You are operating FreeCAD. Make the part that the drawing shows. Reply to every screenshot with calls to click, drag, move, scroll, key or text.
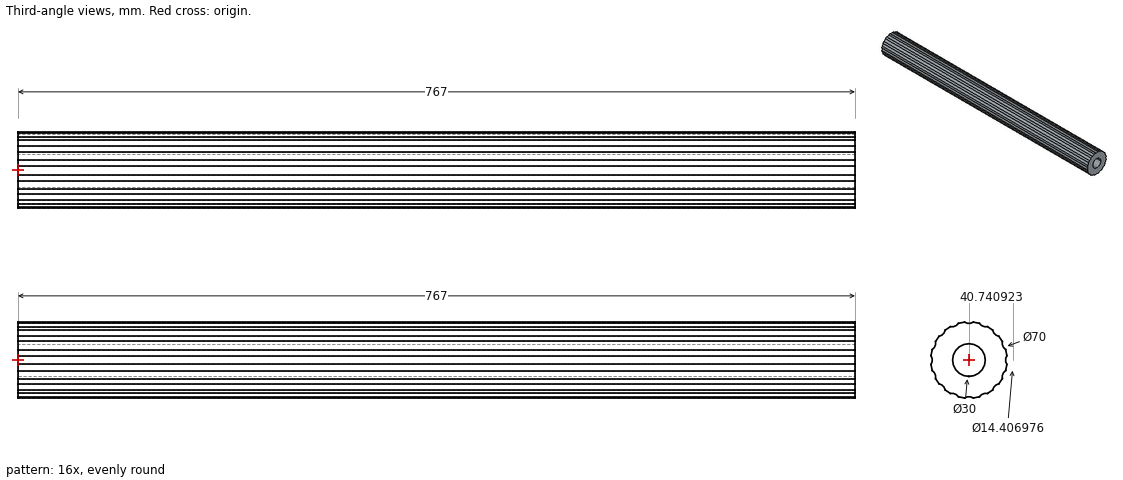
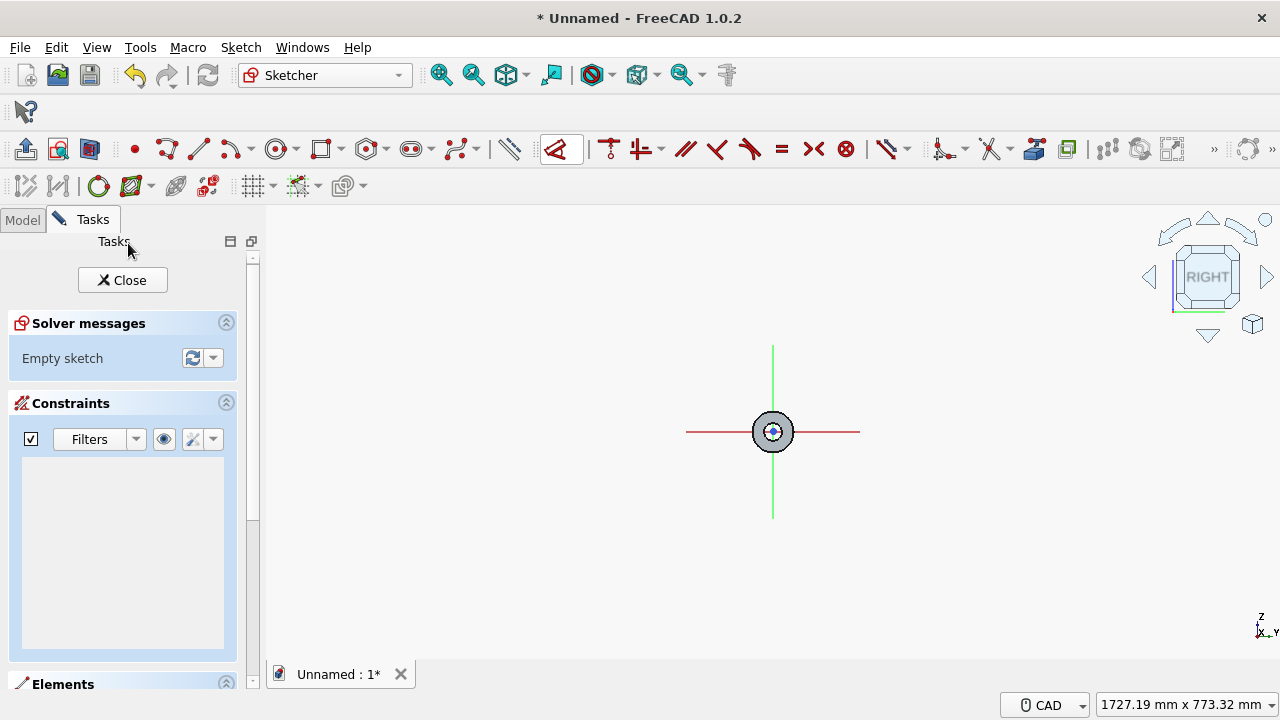
click(90, 150)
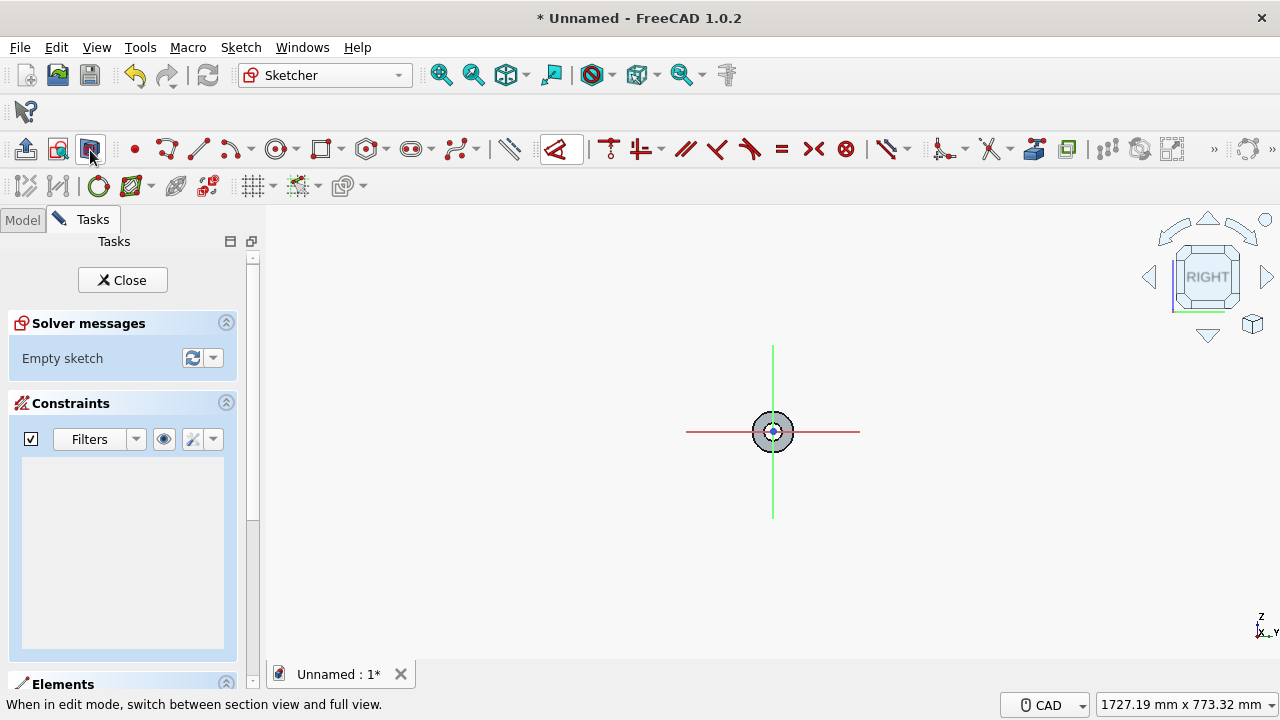
scroll(802, 432, up, 15)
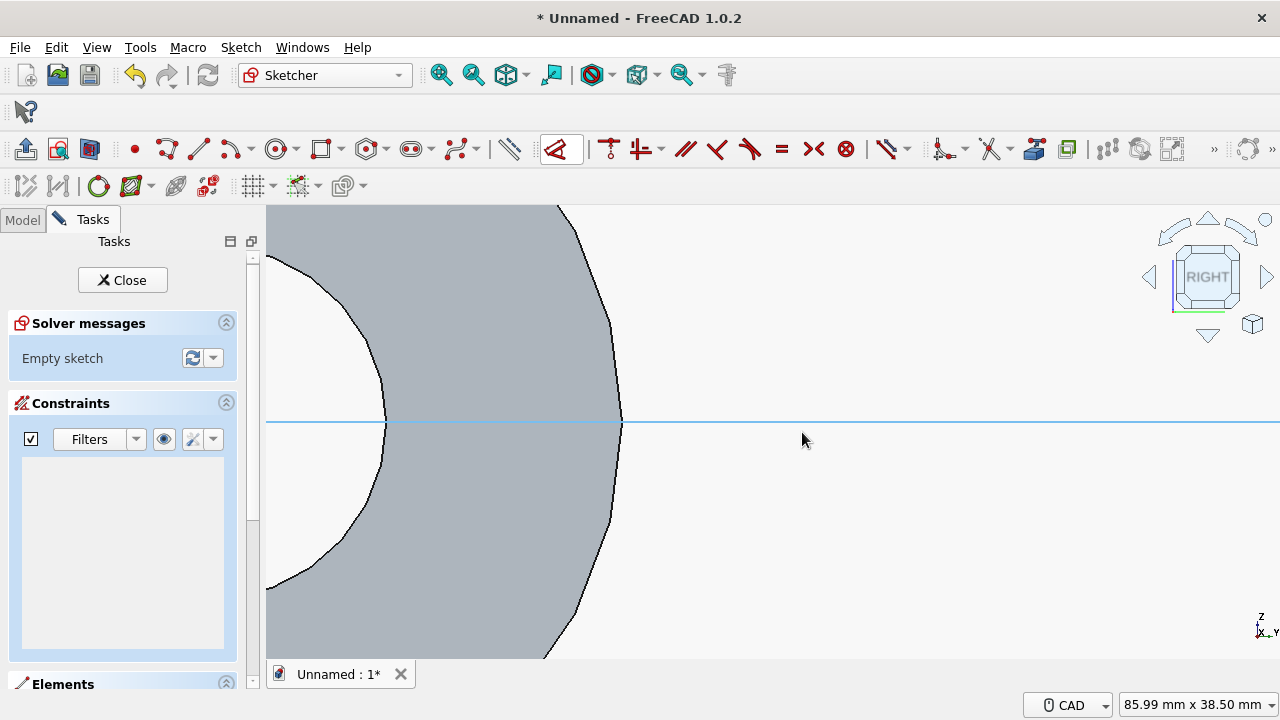
scroll(672, 411, up, 3)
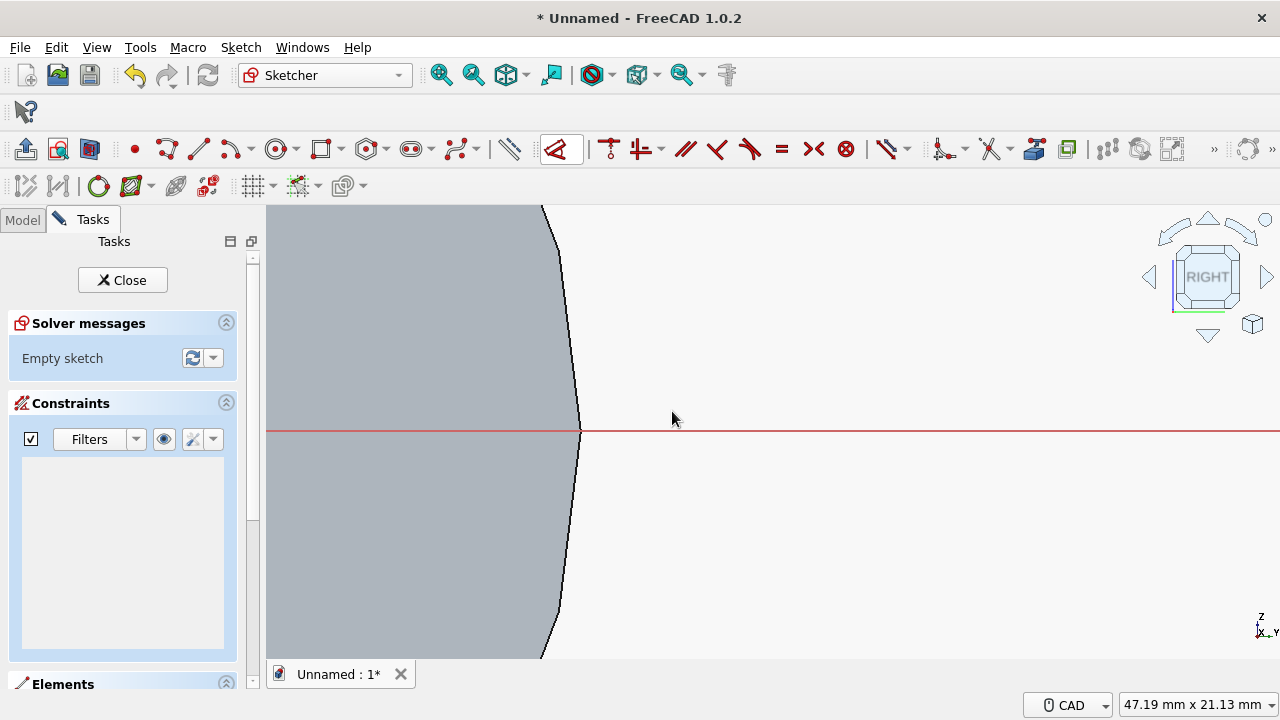
click(276, 150)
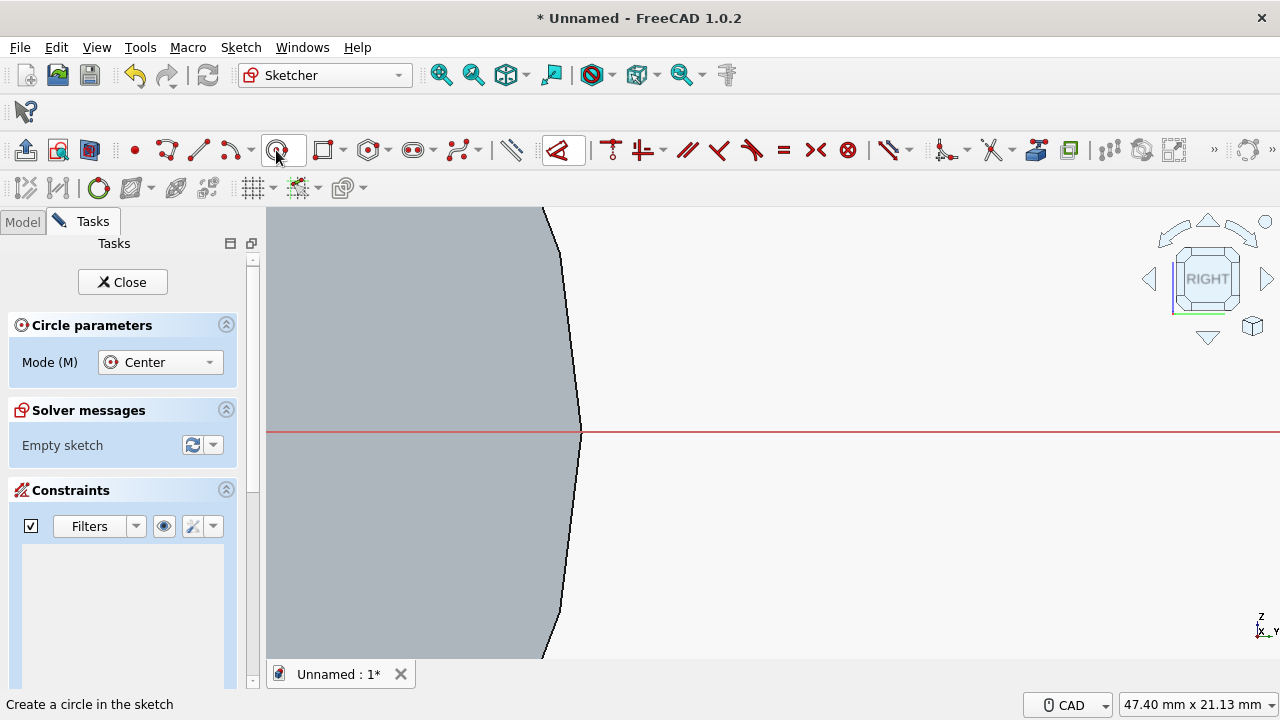
click(704, 432)
click(813, 324)
key(Escape)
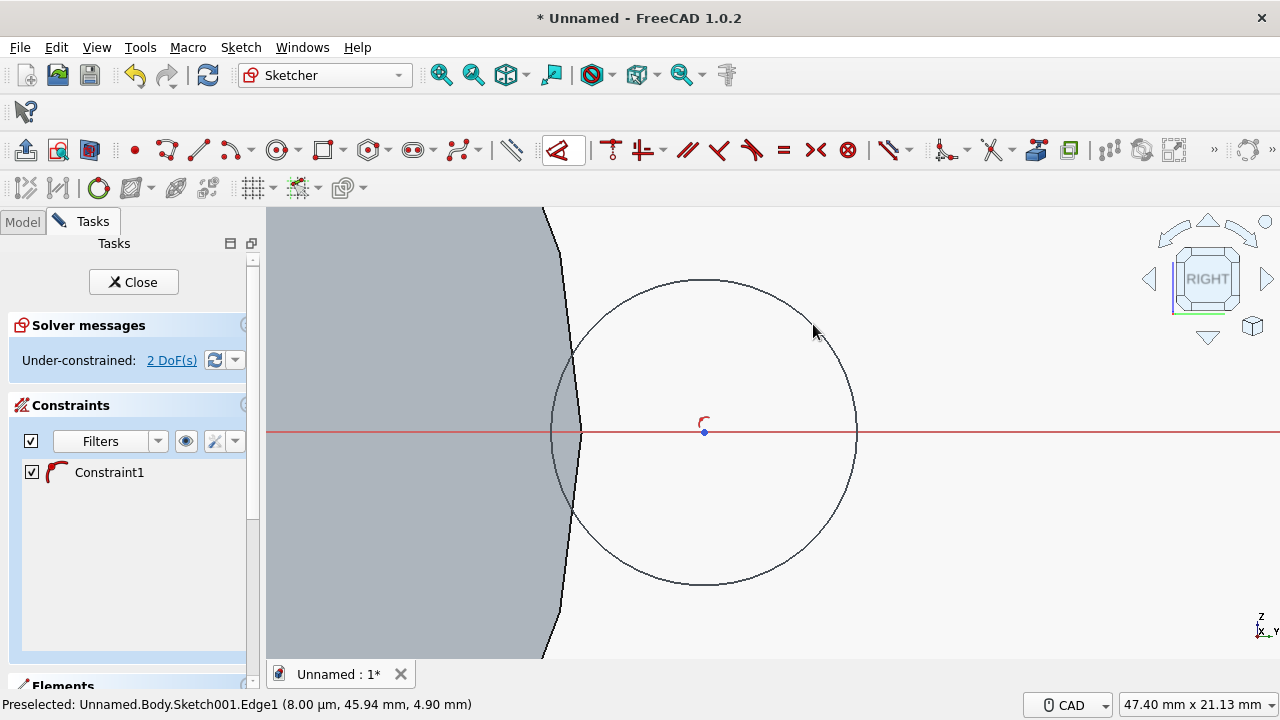
click(812, 324)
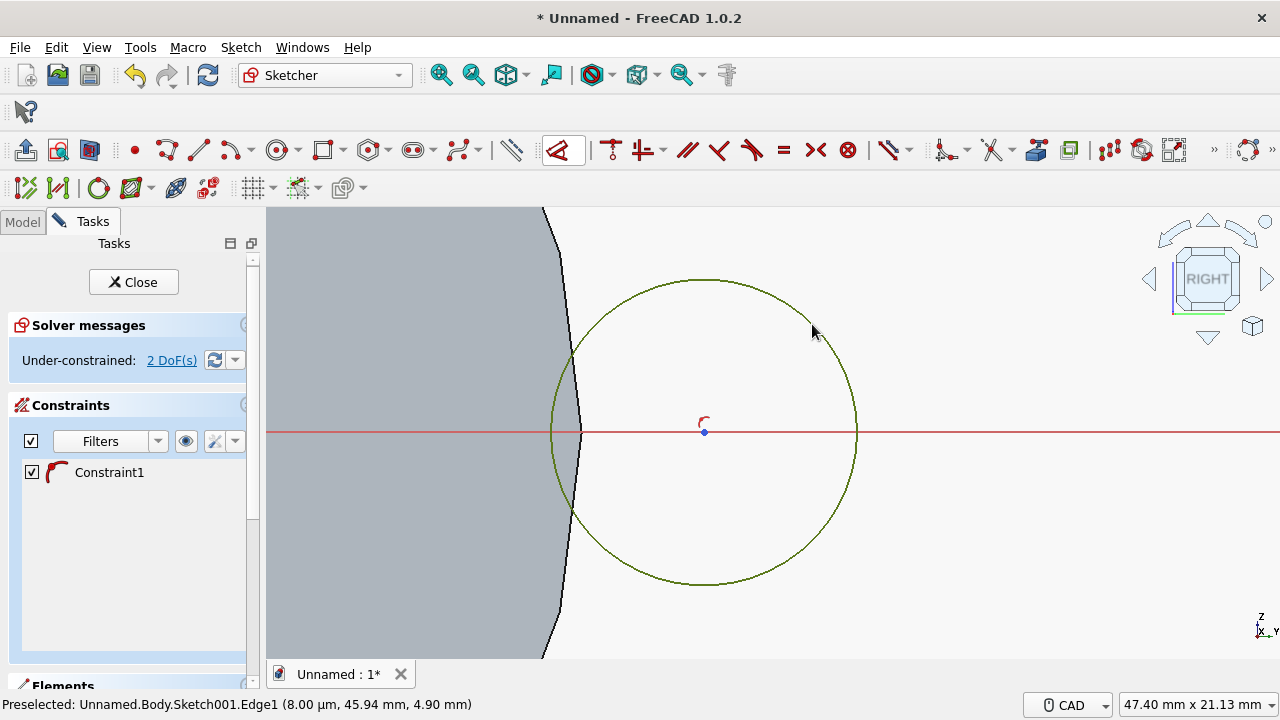
click(580, 150)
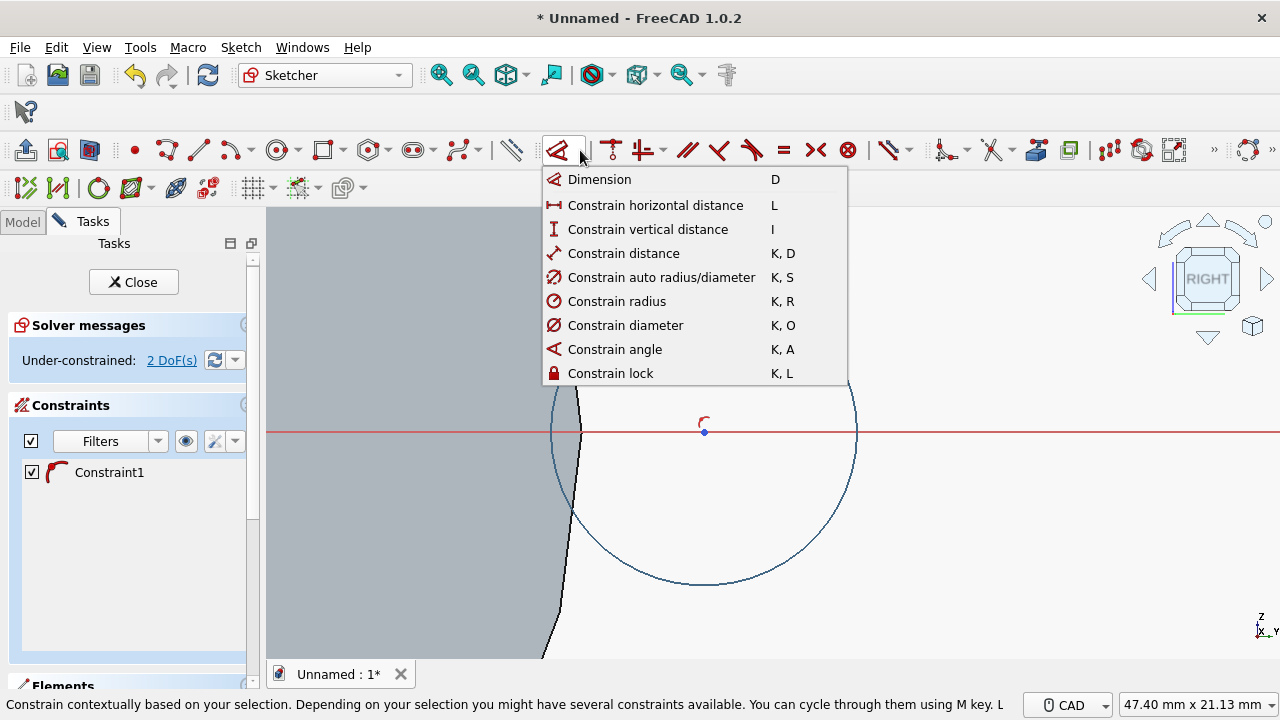
click(695, 325)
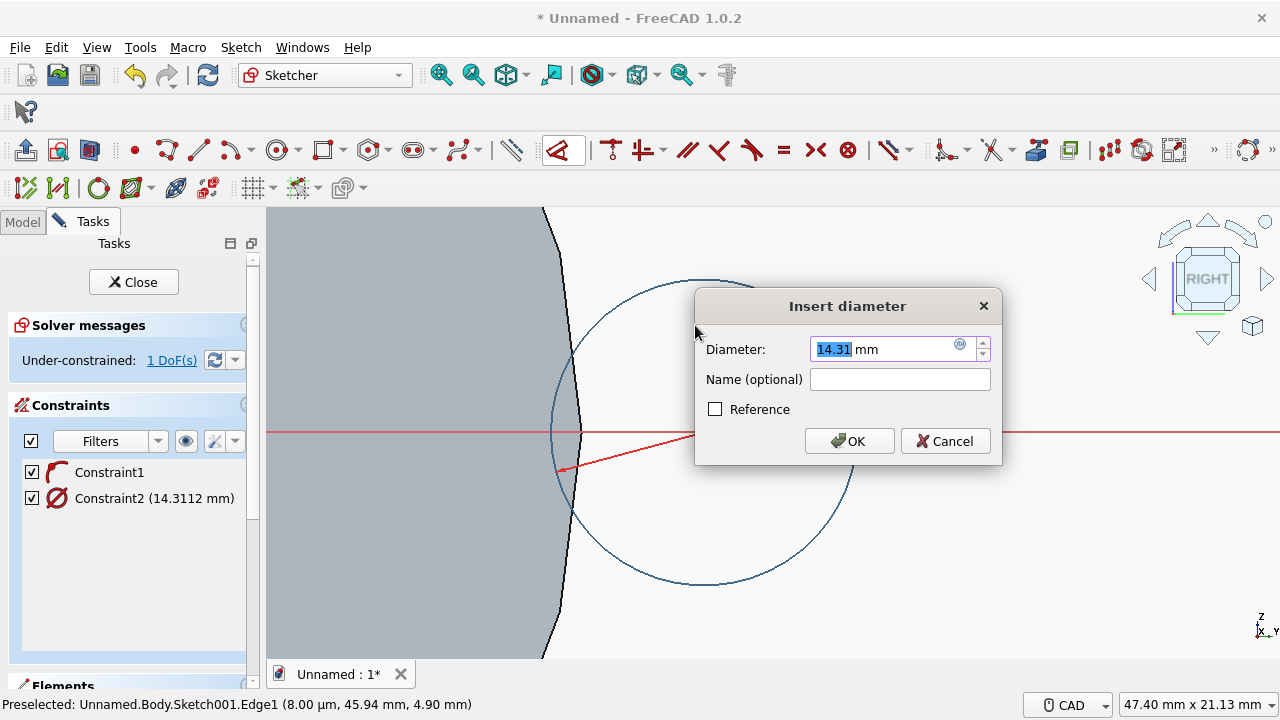
text(14.406976)
key(Return)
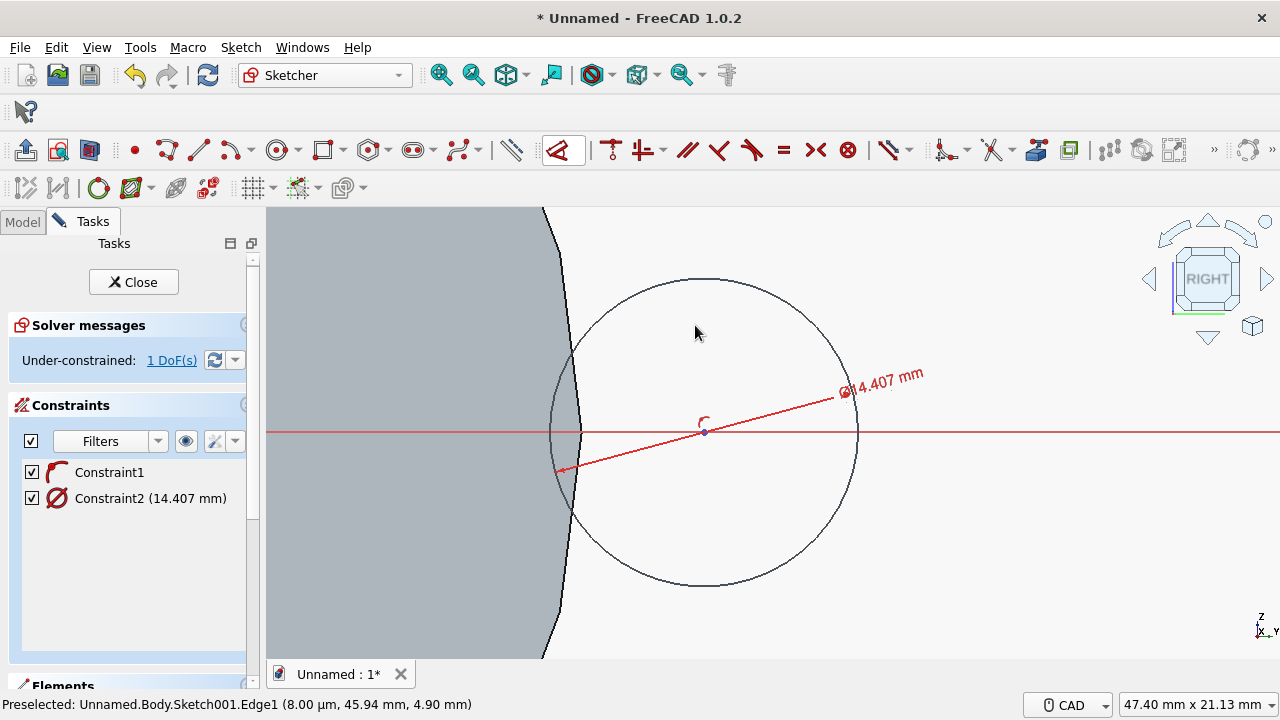
click(704, 432)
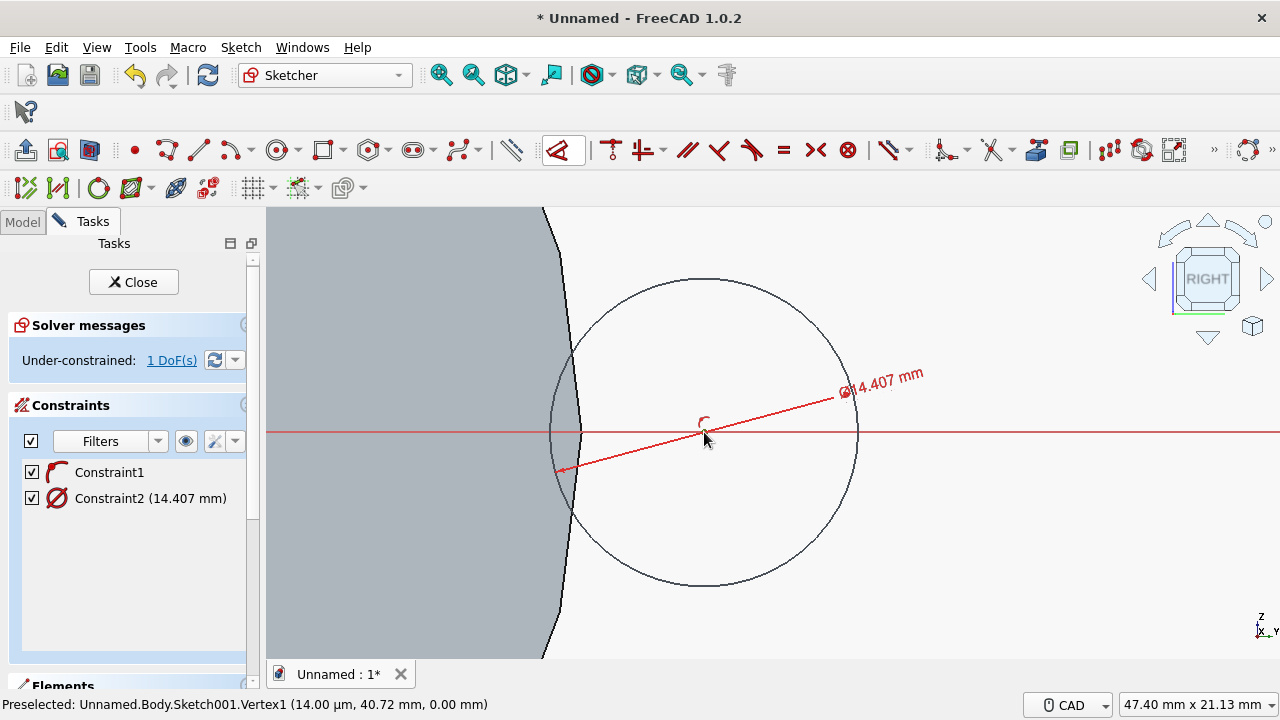
click(580, 150)